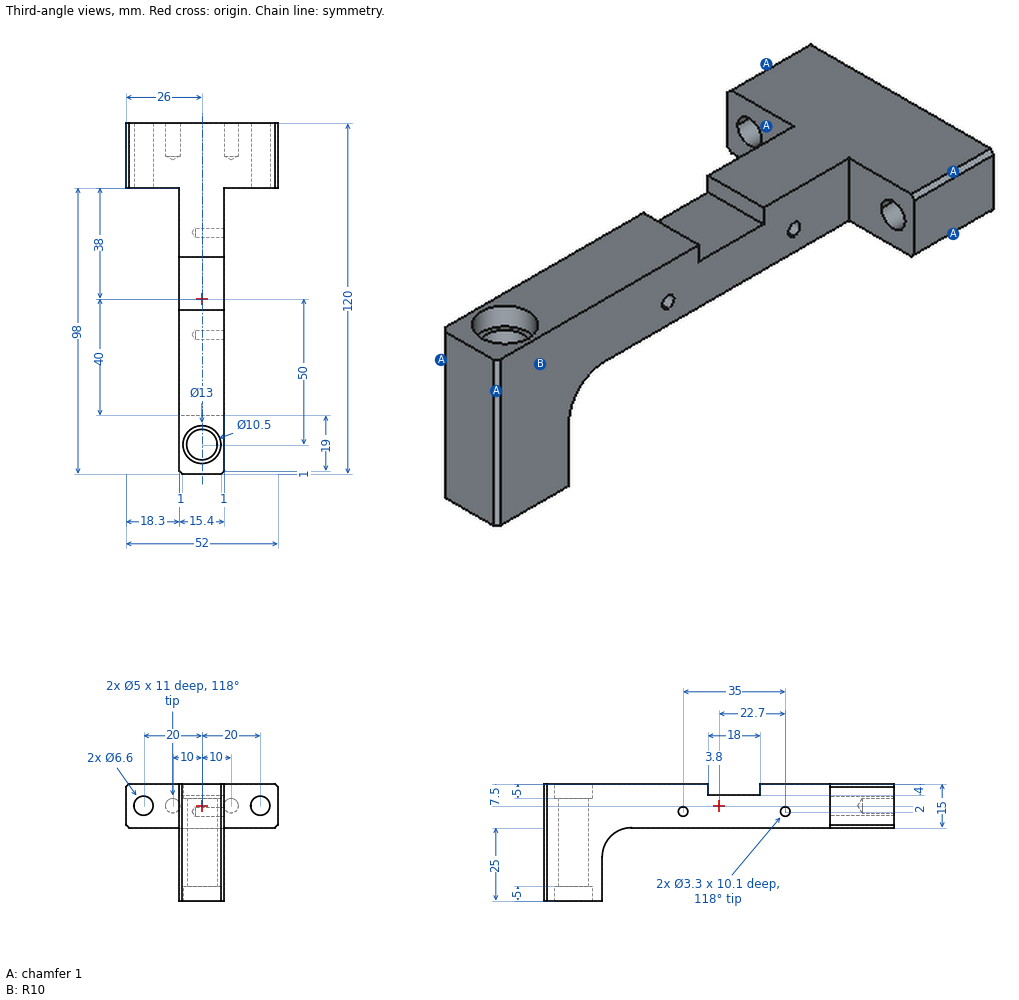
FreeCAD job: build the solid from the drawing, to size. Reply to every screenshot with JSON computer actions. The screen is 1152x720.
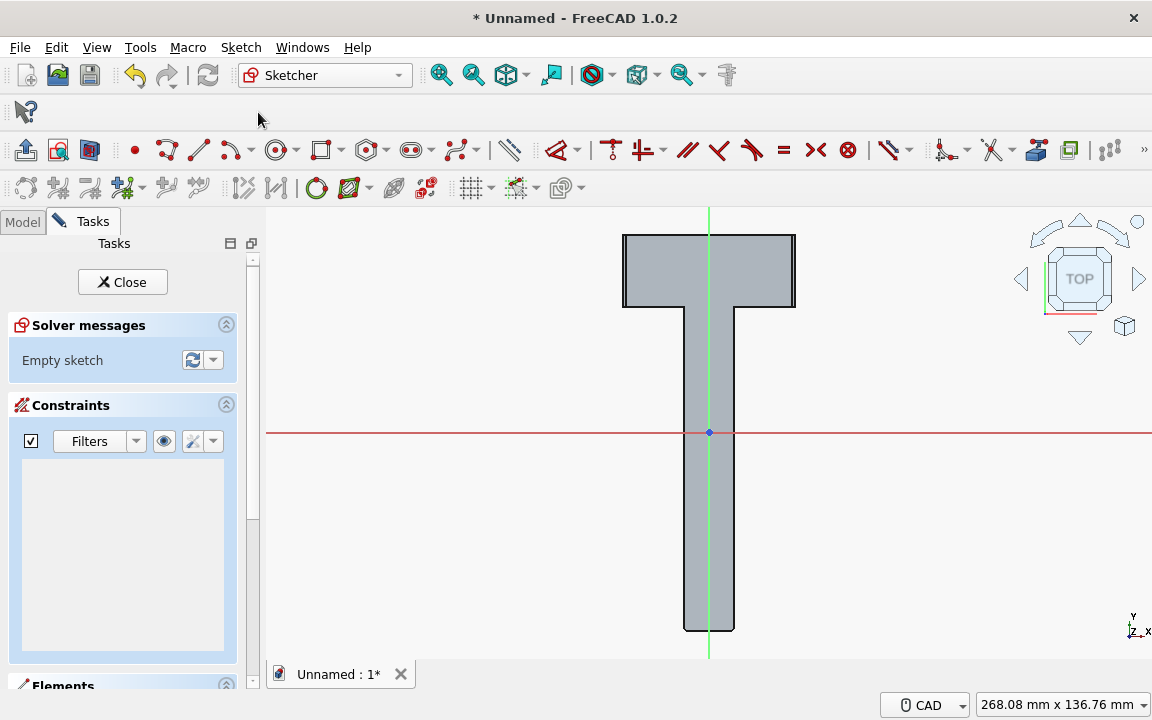
{"action": "scroll", "coordinate": [720, 624], "scroll_direction": "up", "scroll_amount": 10}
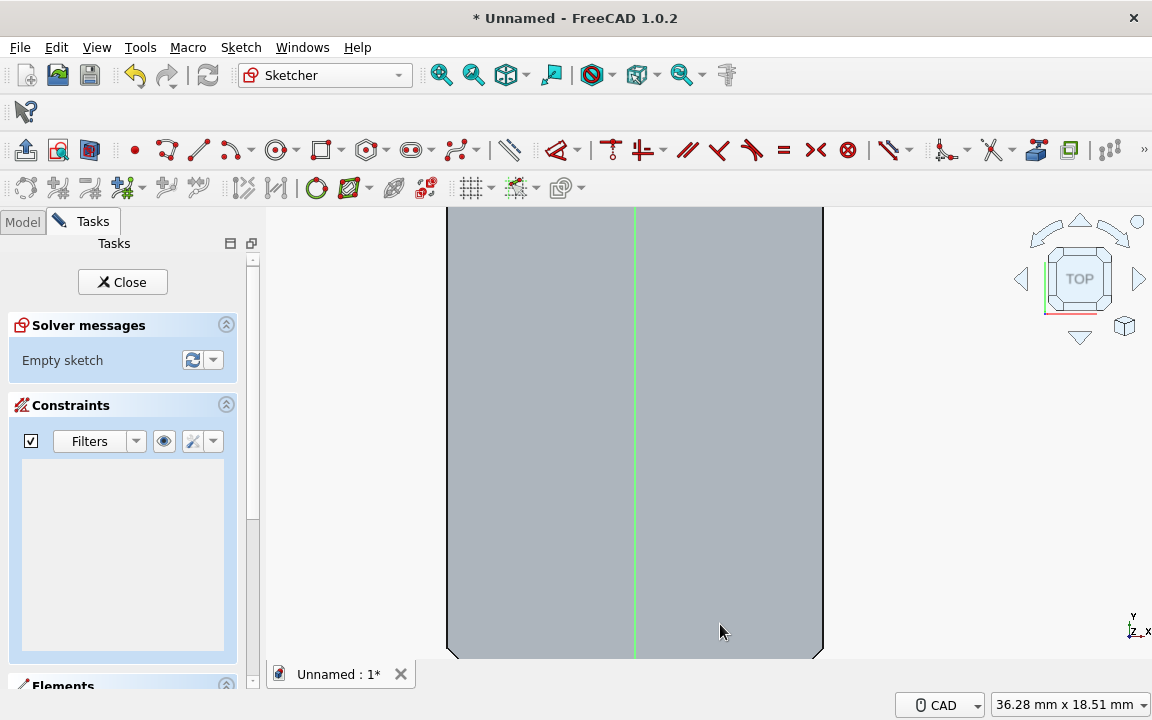
{"action": "left_click", "coordinate": [276, 150]}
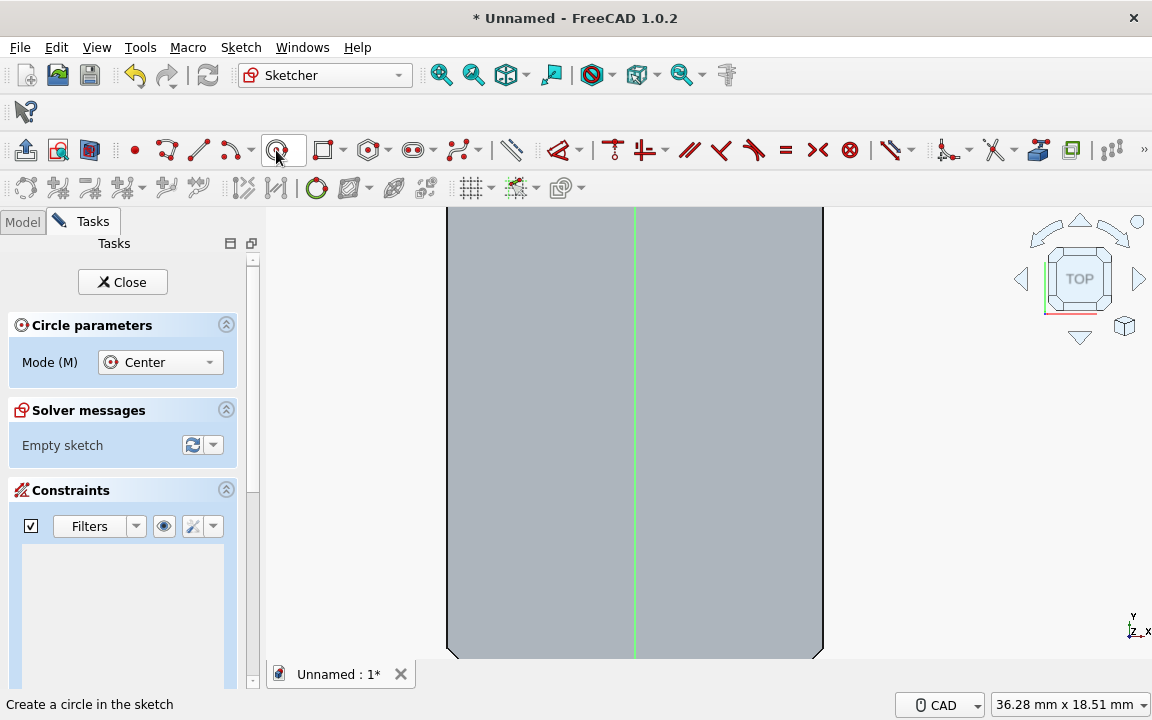
{"action": "left_click", "coordinate": [635, 428]}
{"action": "mouse_move", "coordinate": [726, 337]}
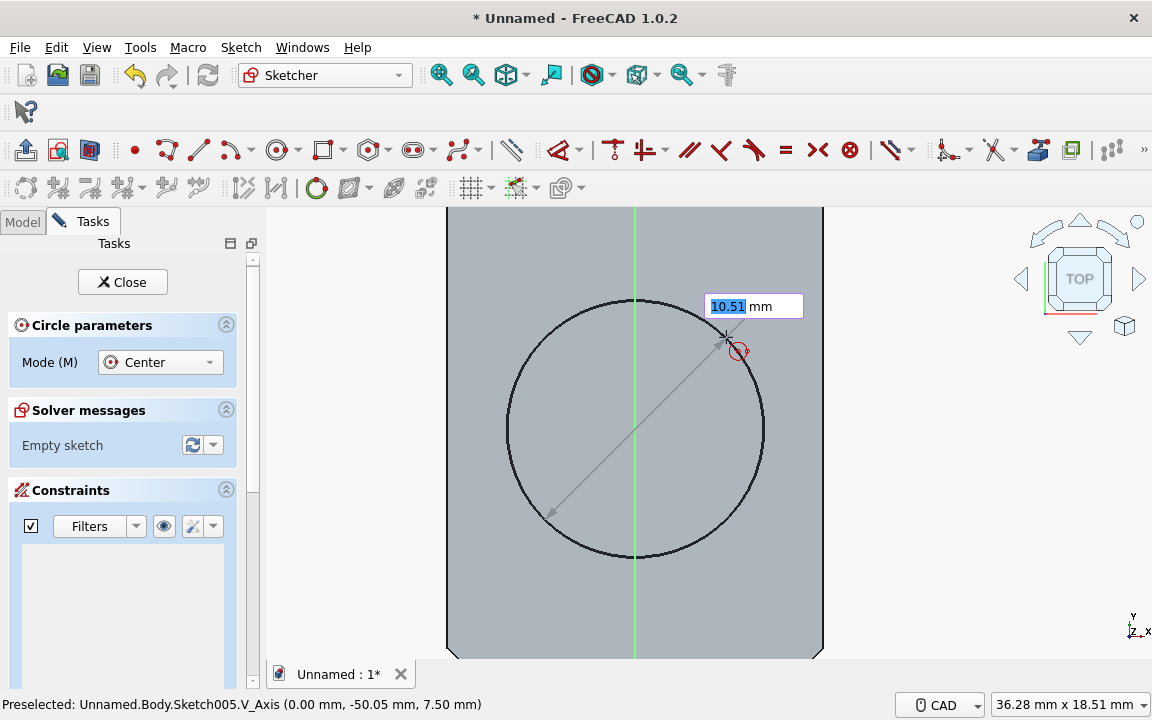
{"action": "type", "text": "10.5"}
{"action": "key", "text": "Return"}
{"action": "key", "text": "Escape"}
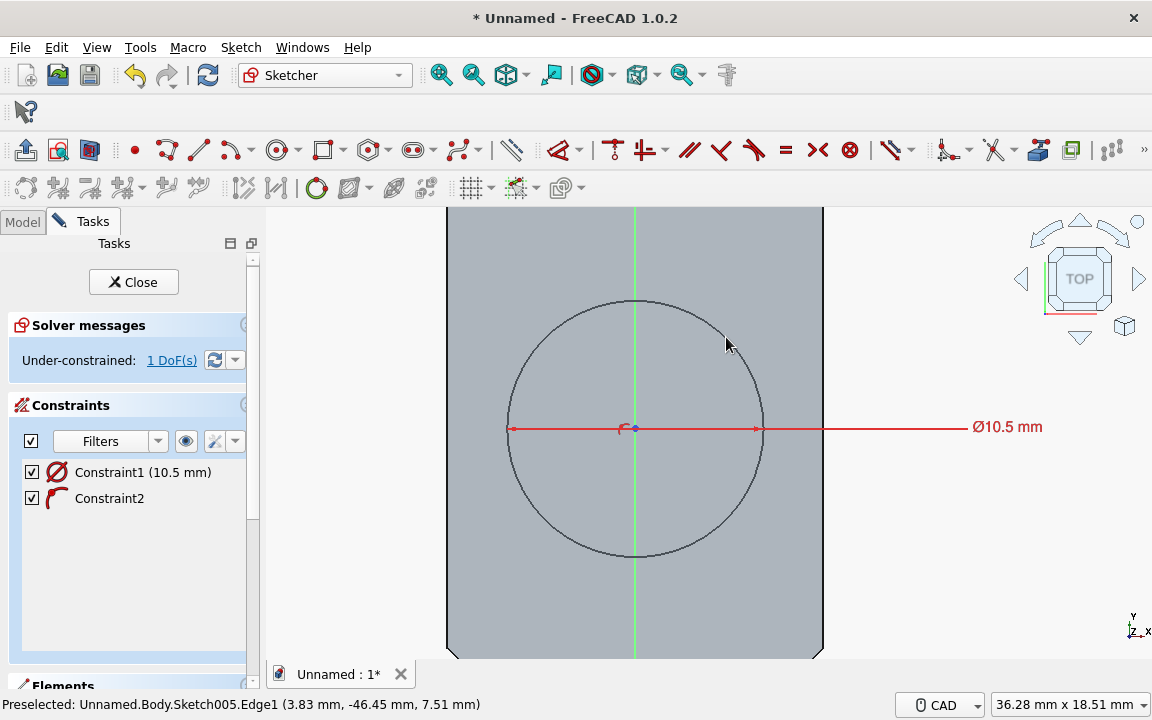
{"action": "left_click", "coordinate": [558, 150]}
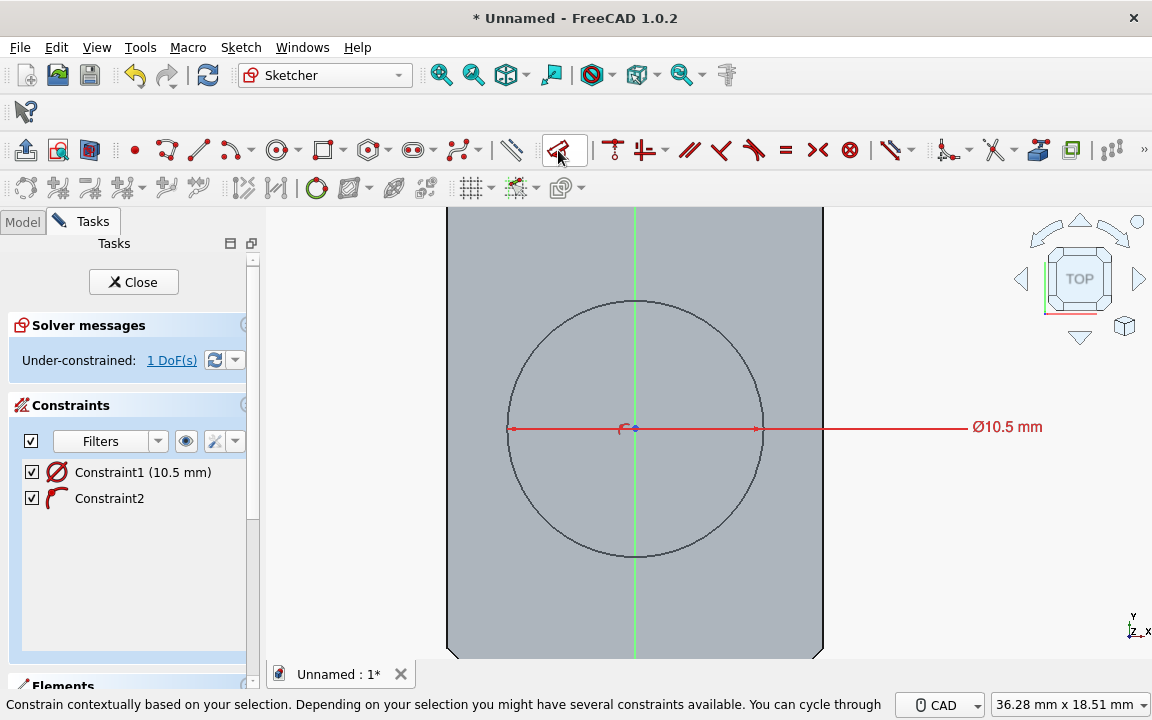
{"action": "left_click", "coordinate": [635, 429]}
{"action": "left_click", "coordinate": [669, 332]}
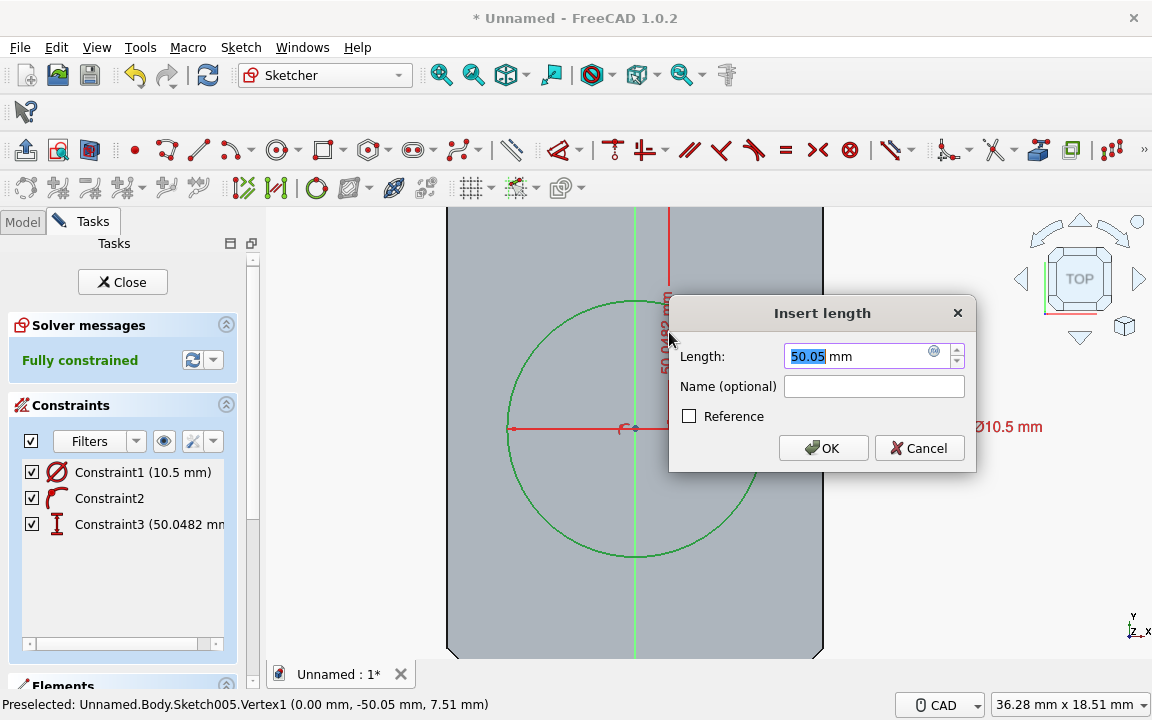
{"action": "type", "text": "50"}
{"action": "key", "text": "Return"}
{"action": "key", "text": "Escape"}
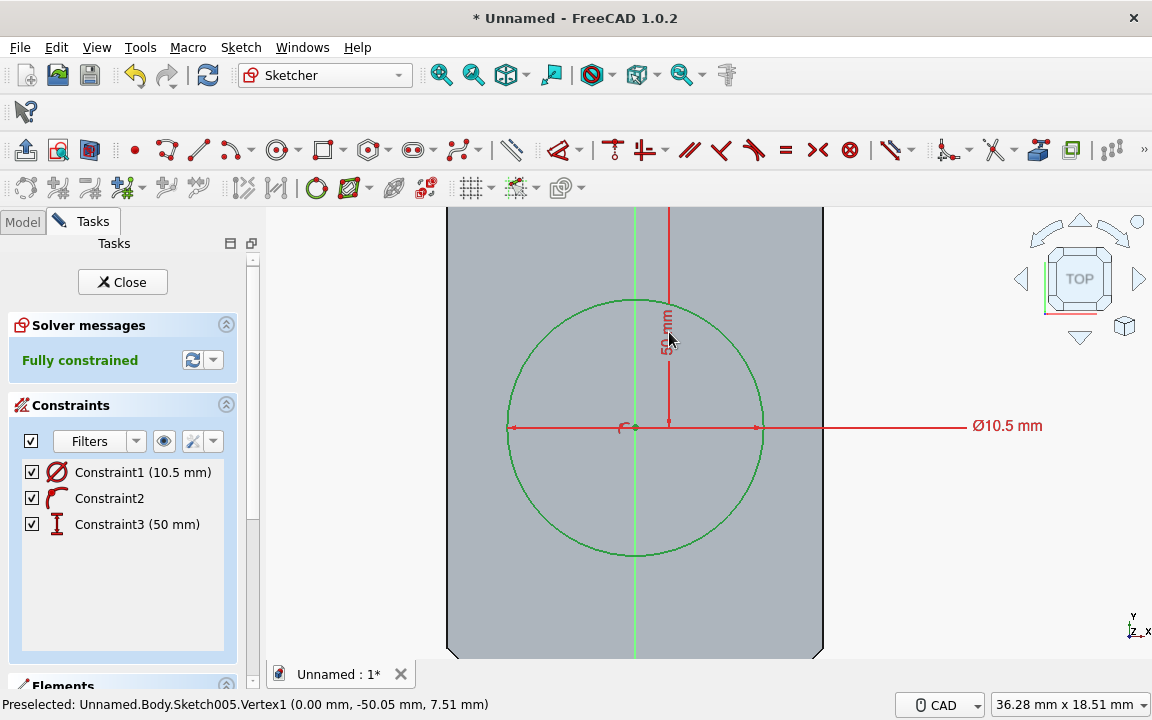
{"action": "left_click", "coordinate": [123, 282]}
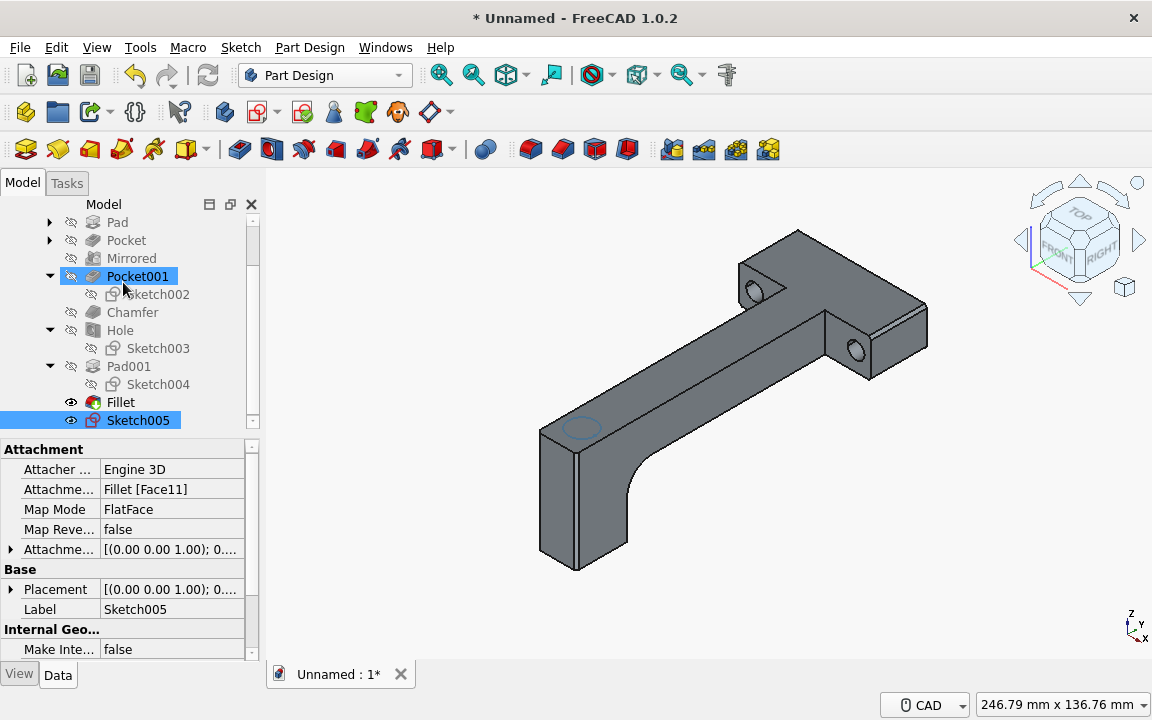
{"action": "left_click", "coordinate": [240, 150]}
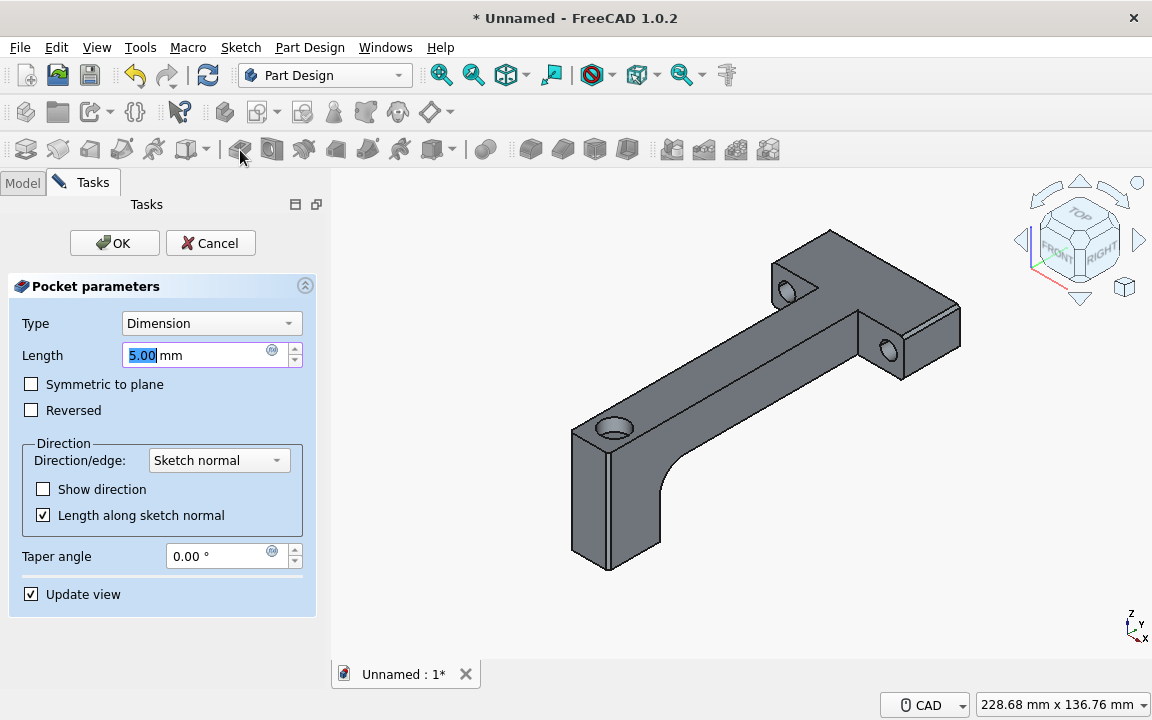
{"action": "left_click", "coordinate": [212, 324]}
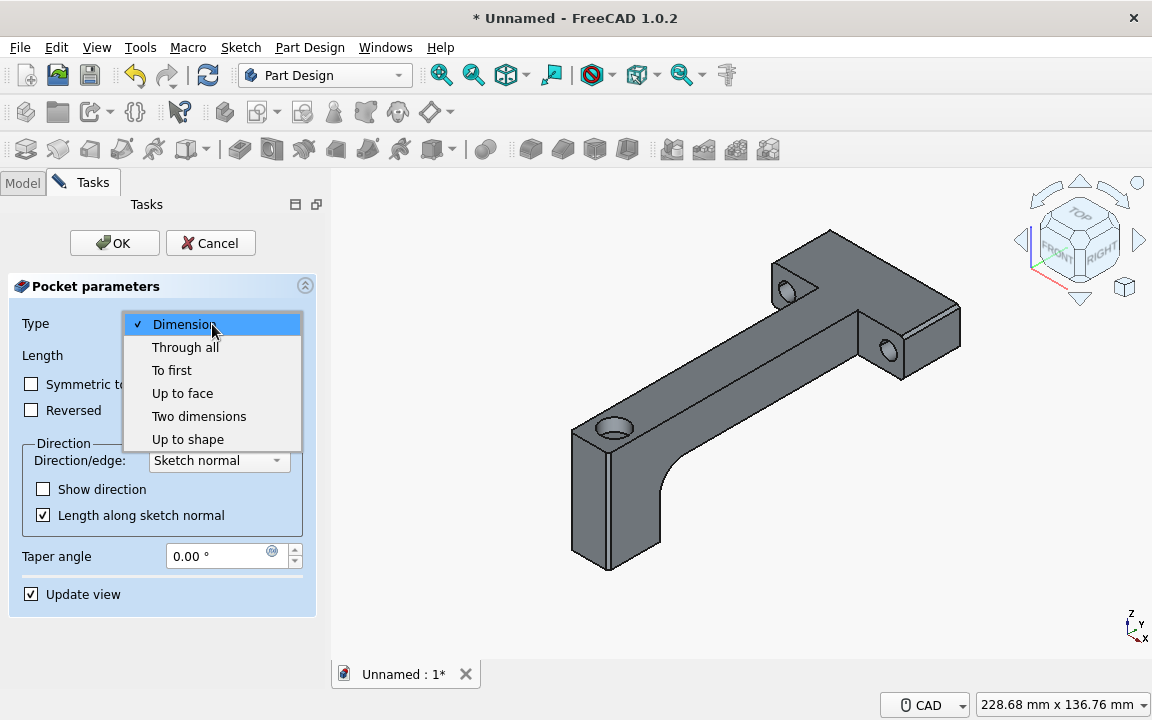
{"action": "left_click", "coordinate": [212, 348]}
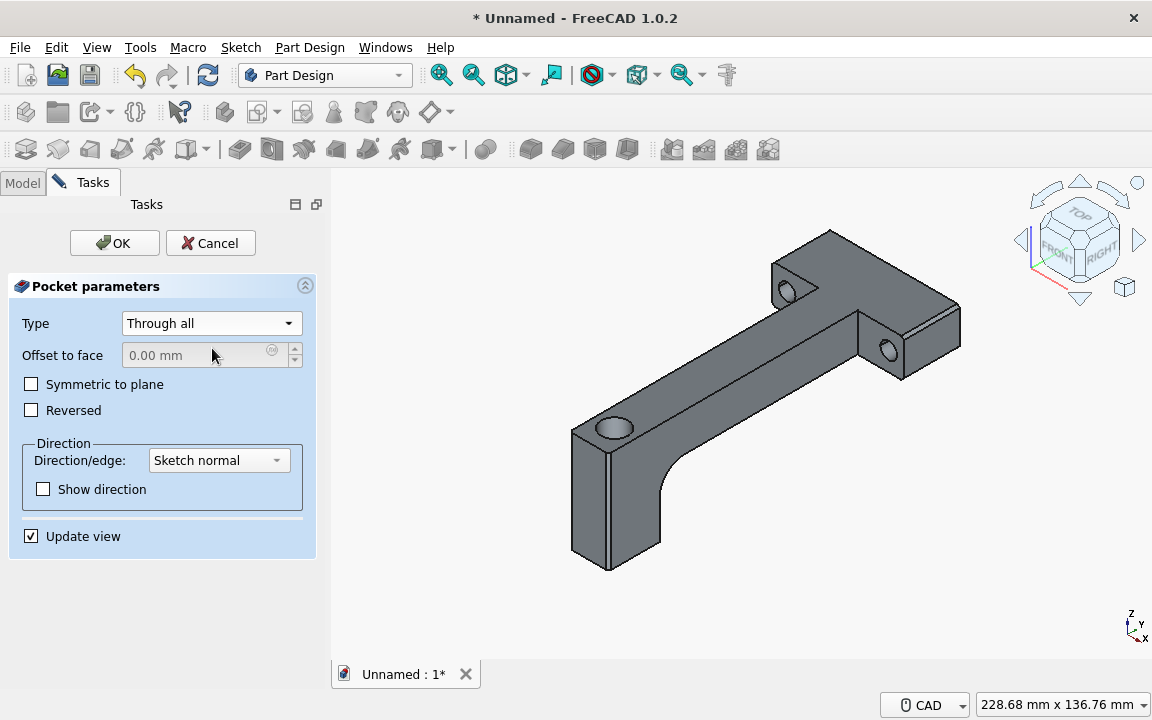
{"action": "left_click", "coordinate": [115, 243]}